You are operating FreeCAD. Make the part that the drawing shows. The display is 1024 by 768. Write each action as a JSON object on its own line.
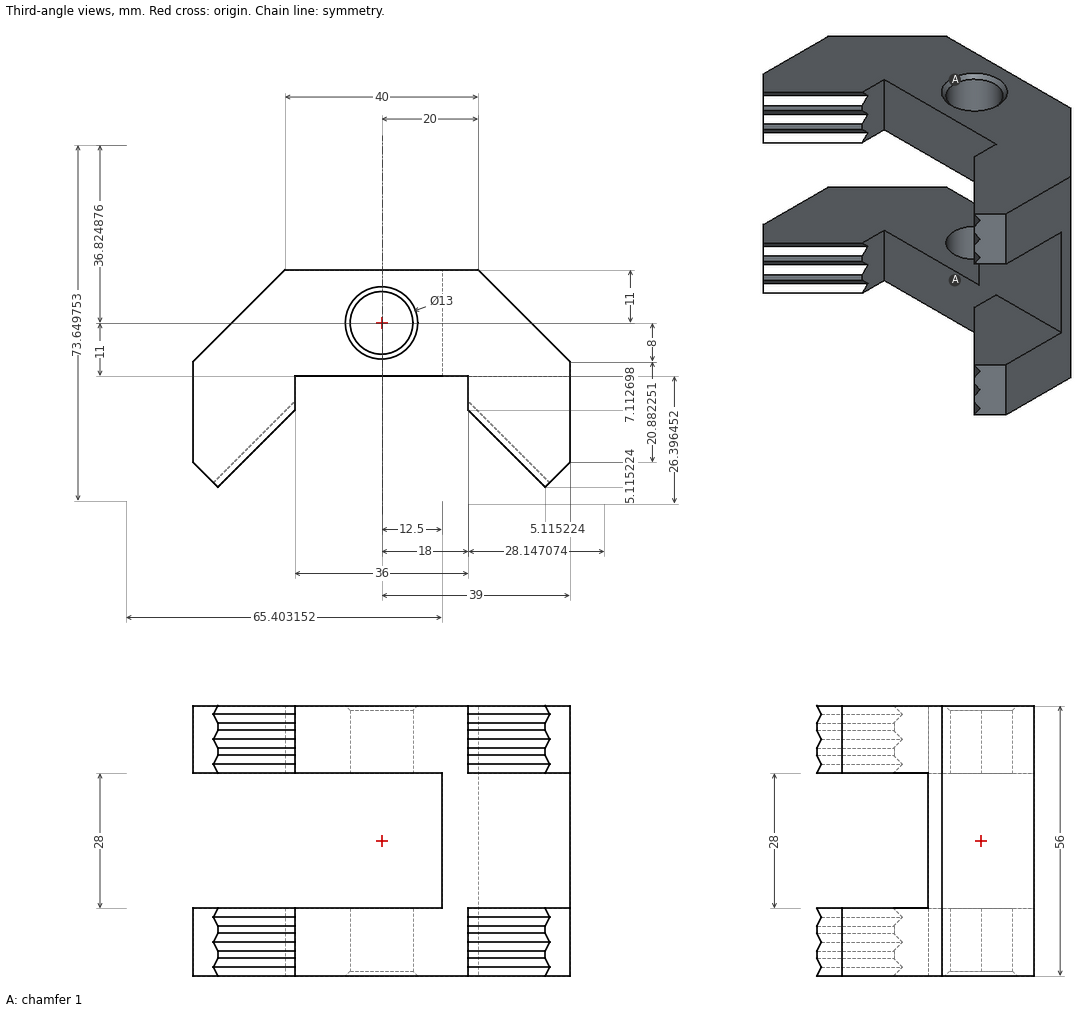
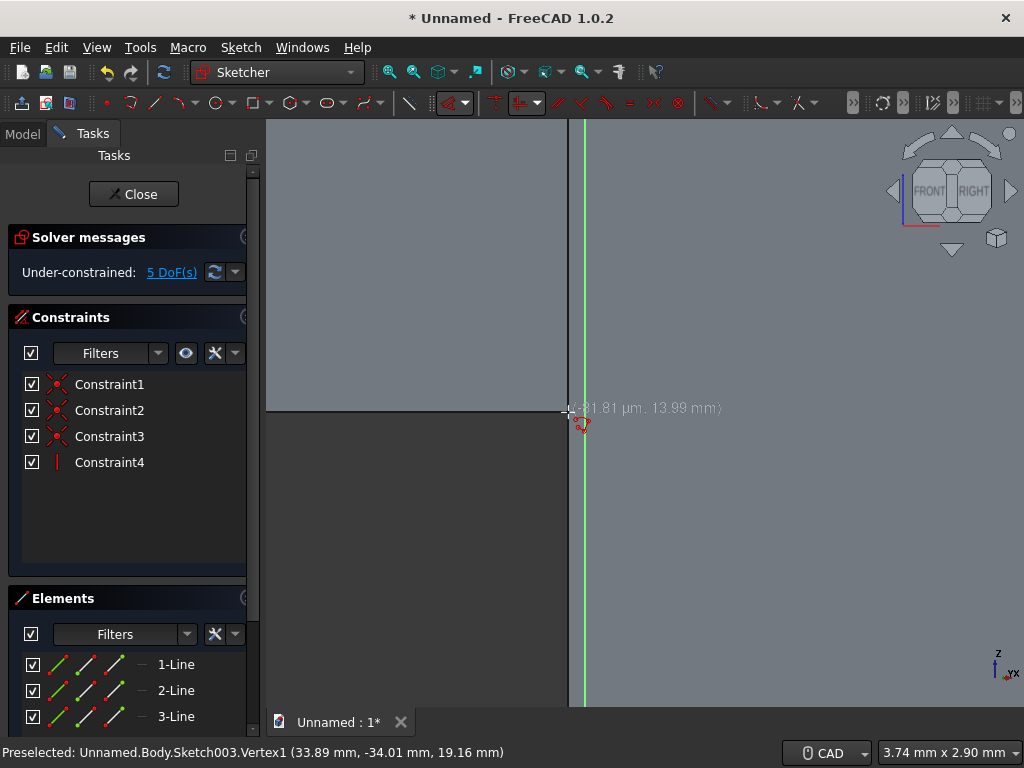
{"action": "scroll", "coordinate": [569, 413], "scroll_direction": "down", "scroll_amount": 14}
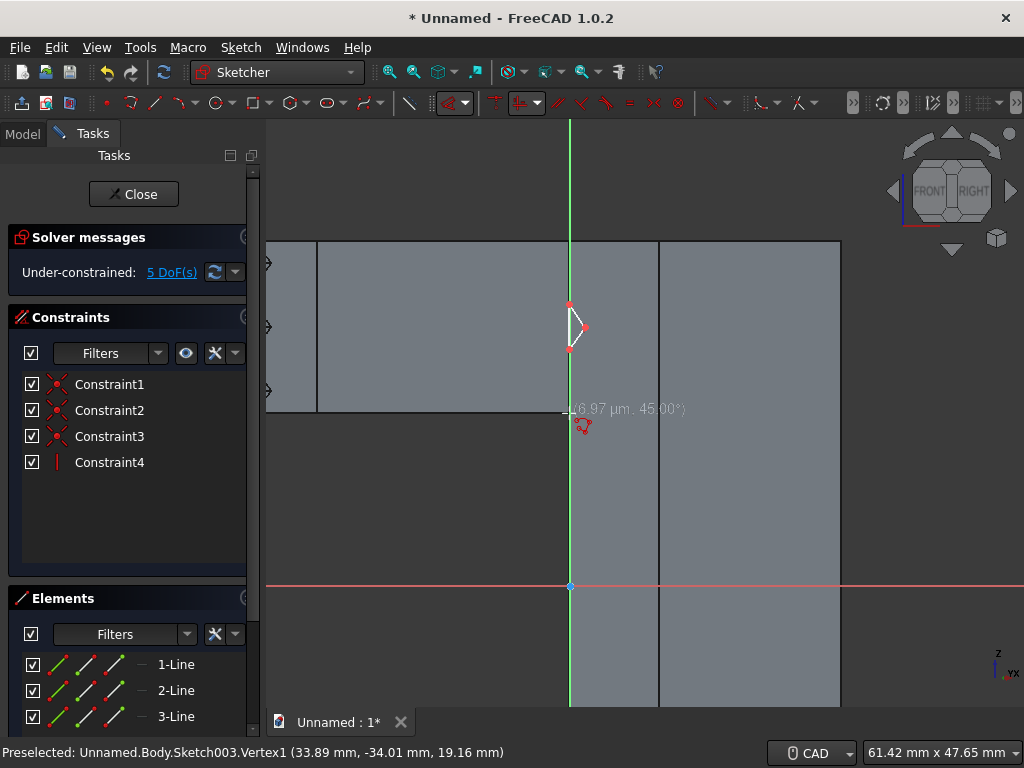
{"action": "left_click", "coordinate": [585, 391]}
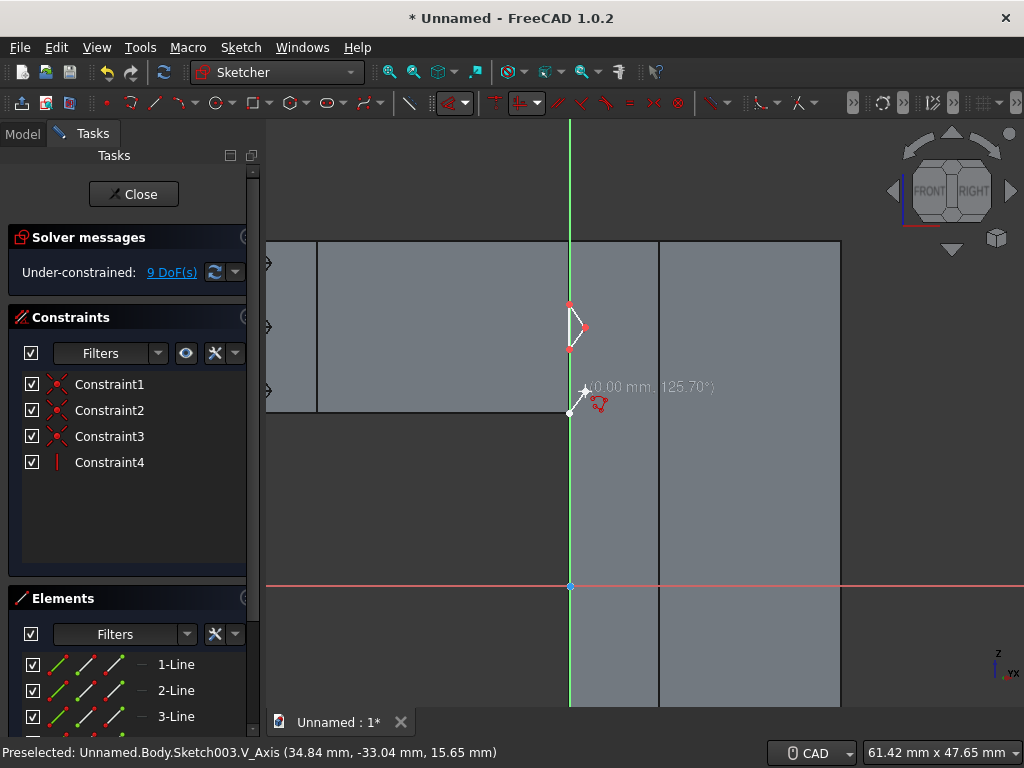
{"action": "scroll", "coordinate": [569, 368], "scroll_direction": "up", "scroll_amount": 14}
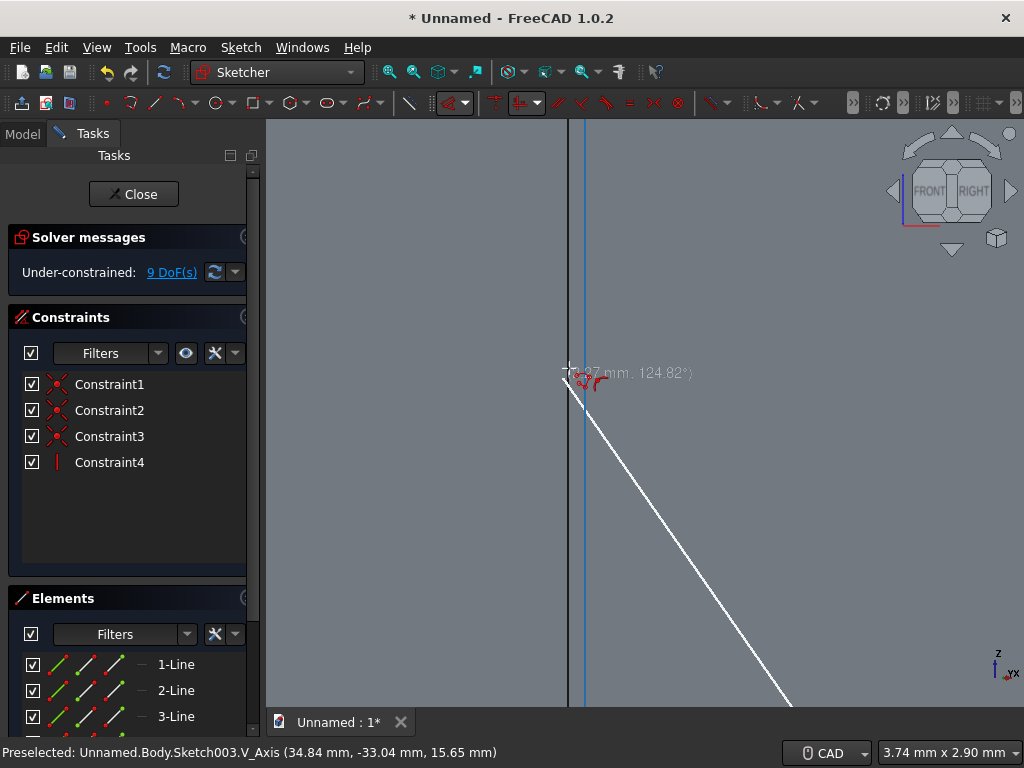
{"action": "left_click", "coordinate": [568, 364]}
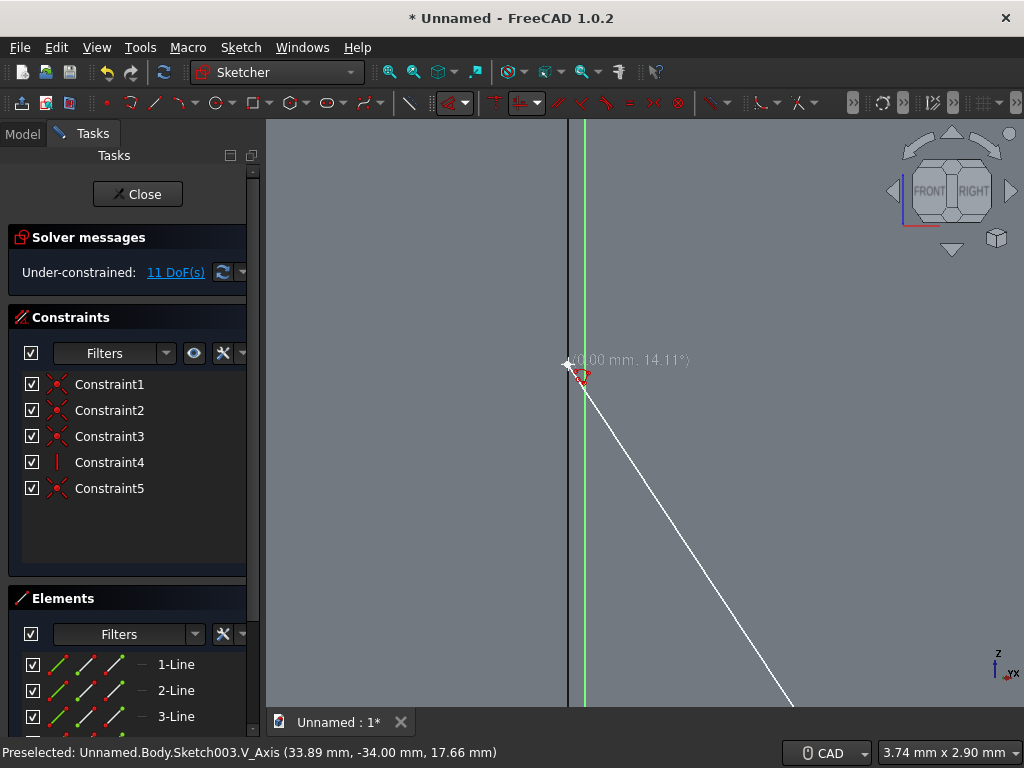
{"action": "scroll", "coordinate": [569, 368], "scroll_direction": "down", "scroll_amount": 14}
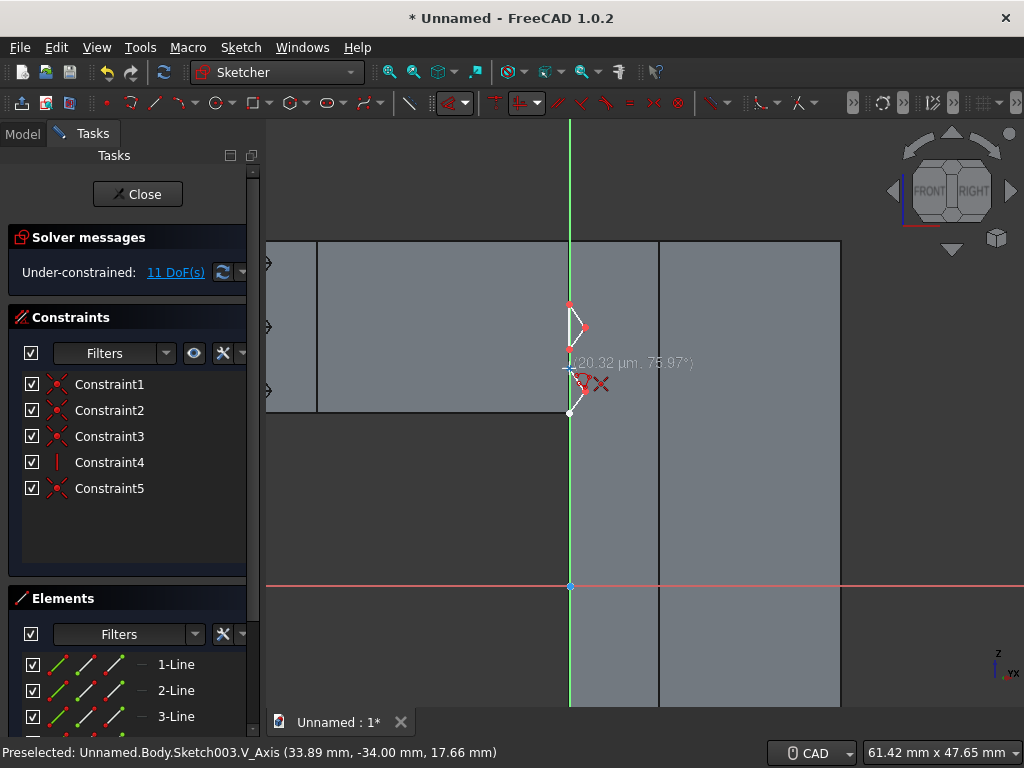
{"action": "scroll", "coordinate": [569, 413], "scroll_direction": "up", "scroll_amount": 14}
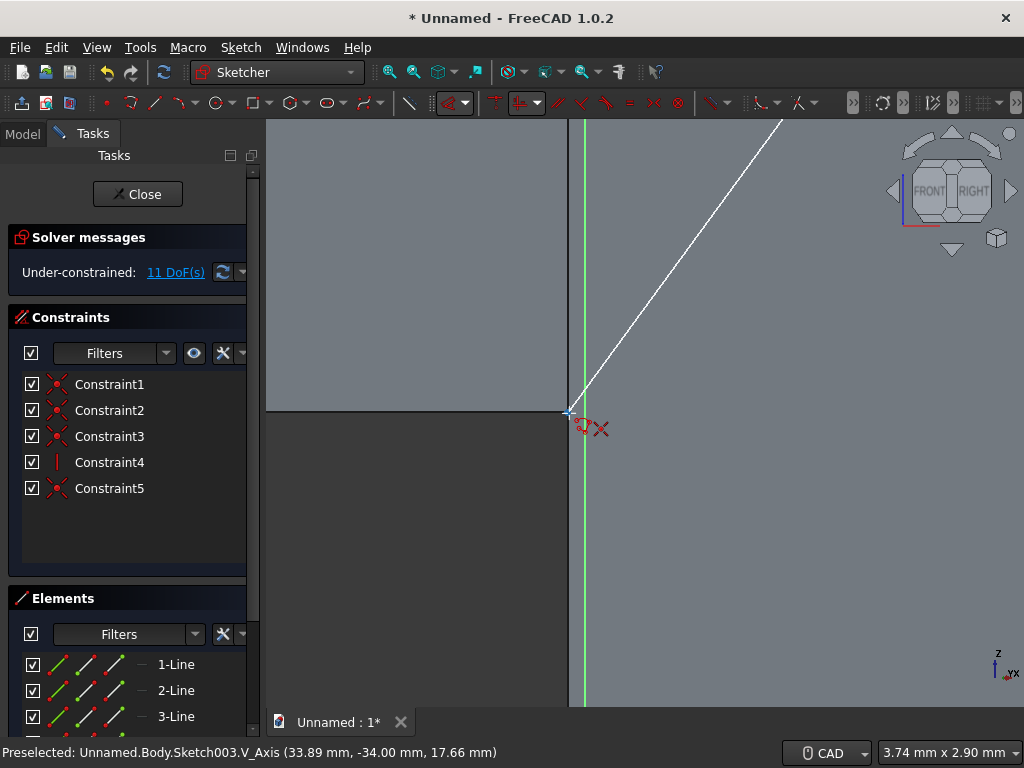
{"action": "left_click", "coordinate": [568, 413]}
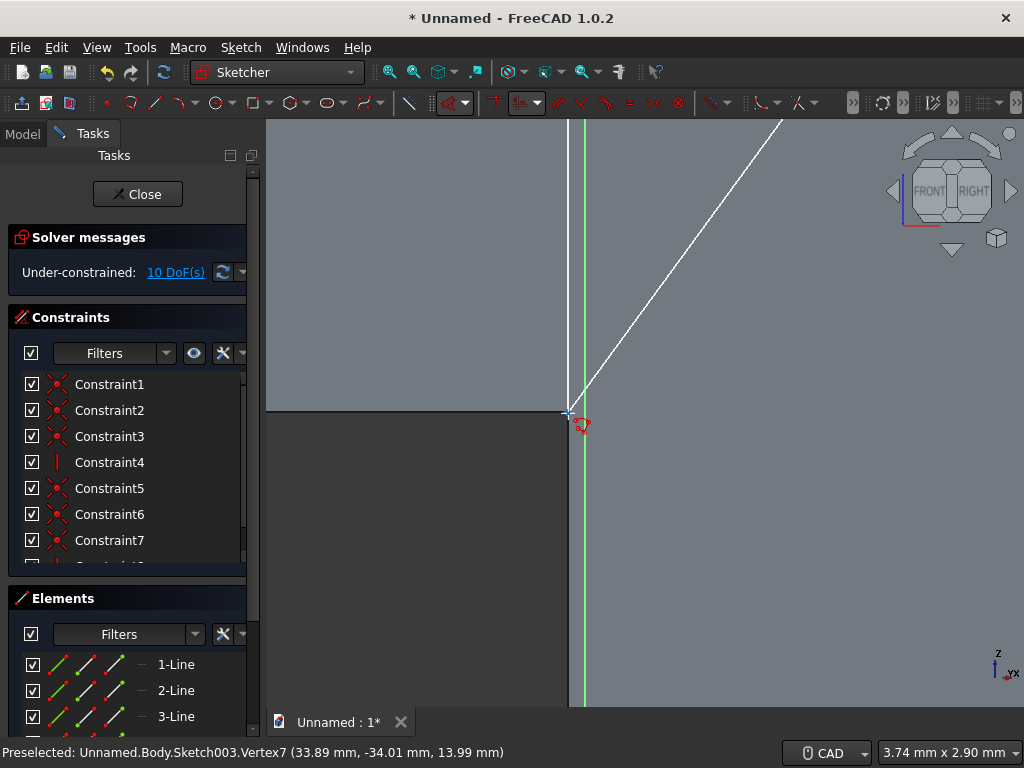
{"action": "scroll", "coordinate": [569, 413], "scroll_direction": "down", "scroll_amount": 14}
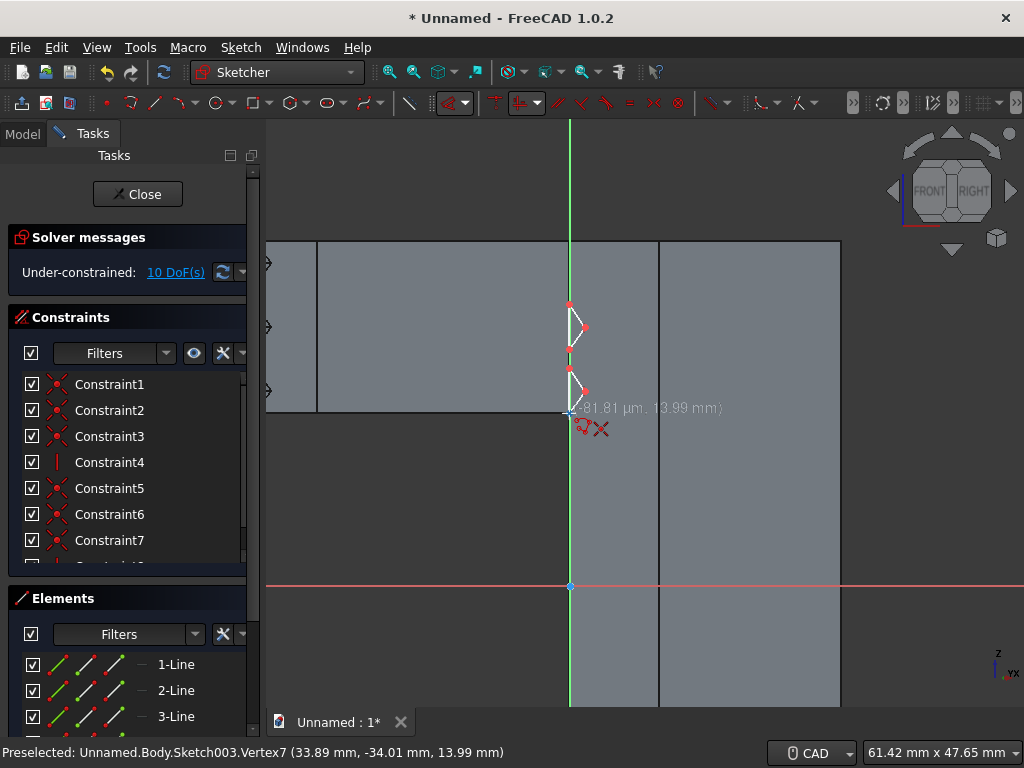
{"action": "scroll", "coordinate": [569, 286], "scroll_direction": "up", "scroll_amount": 14}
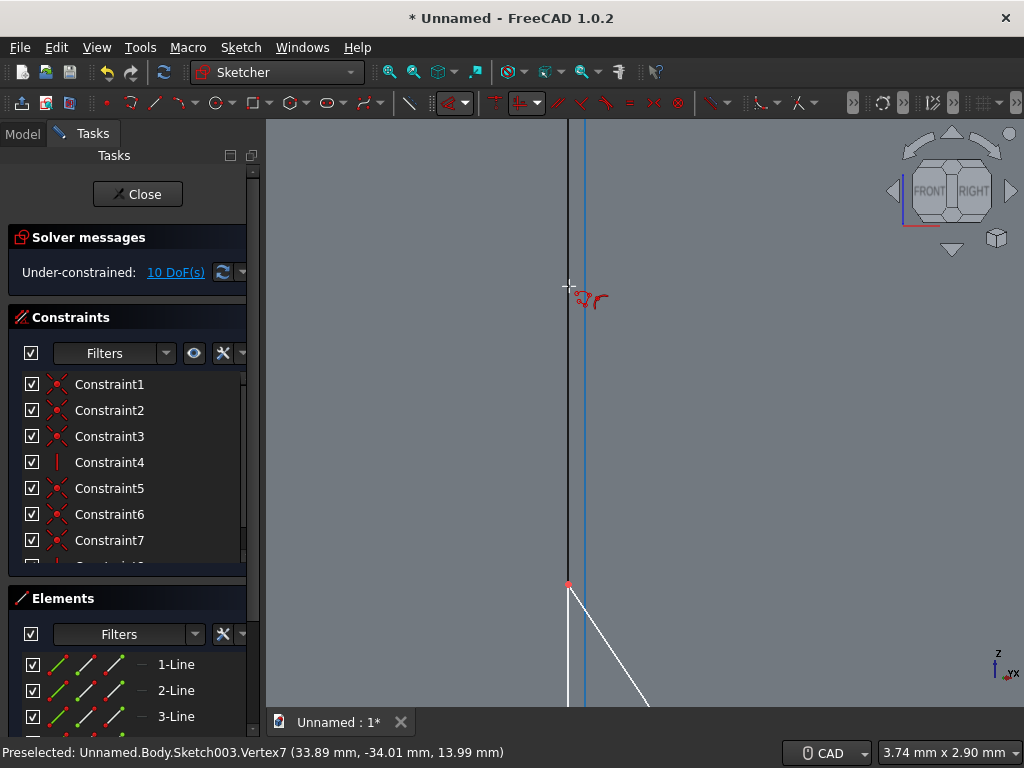
{"action": "left_click", "coordinate": [568, 279]}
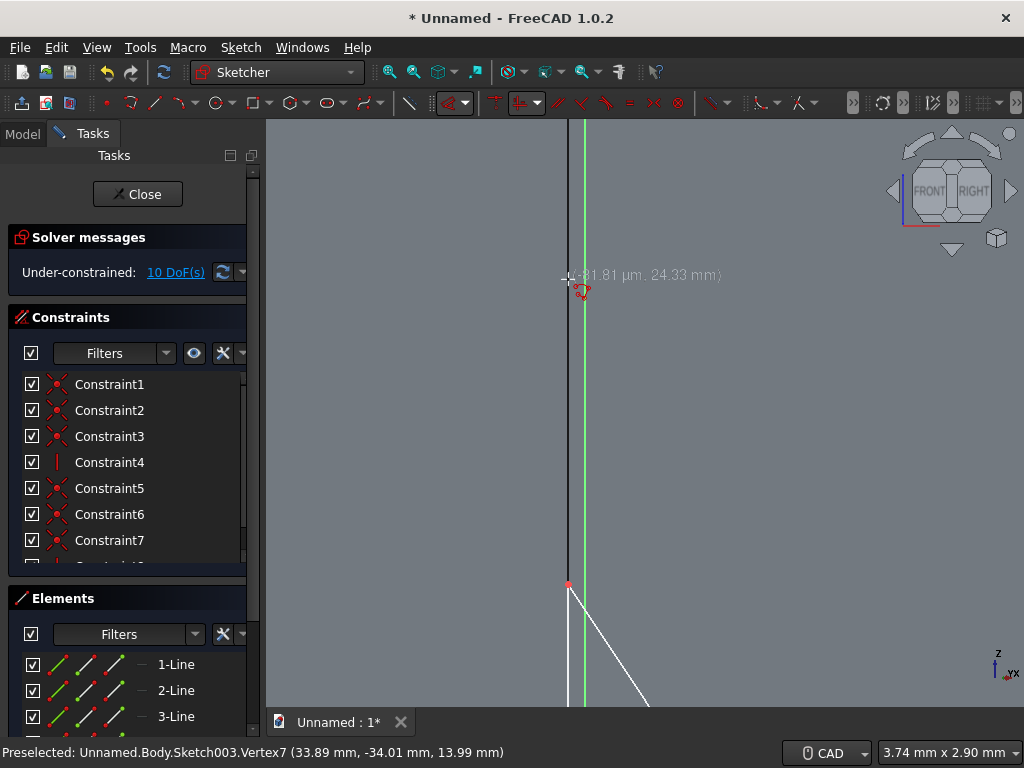
{"action": "scroll", "coordinate": [569, 286], "scroll_direction": "down", "scroll_amount": 14}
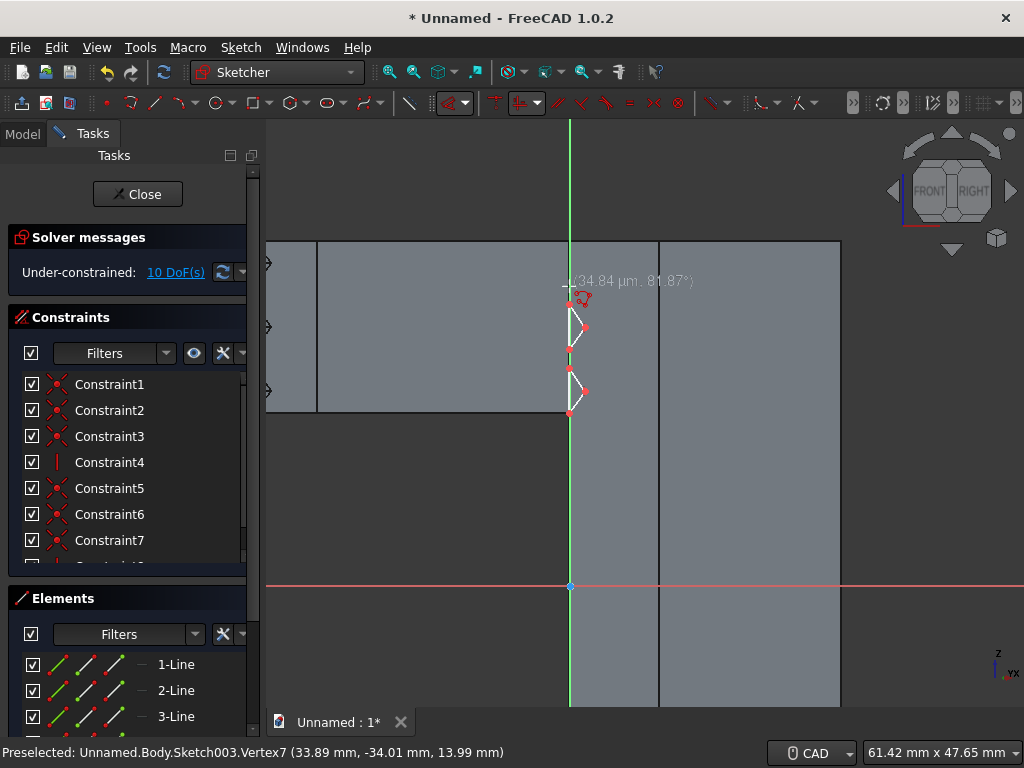
{"action": "left_click", "coordinate": [585, 263]}